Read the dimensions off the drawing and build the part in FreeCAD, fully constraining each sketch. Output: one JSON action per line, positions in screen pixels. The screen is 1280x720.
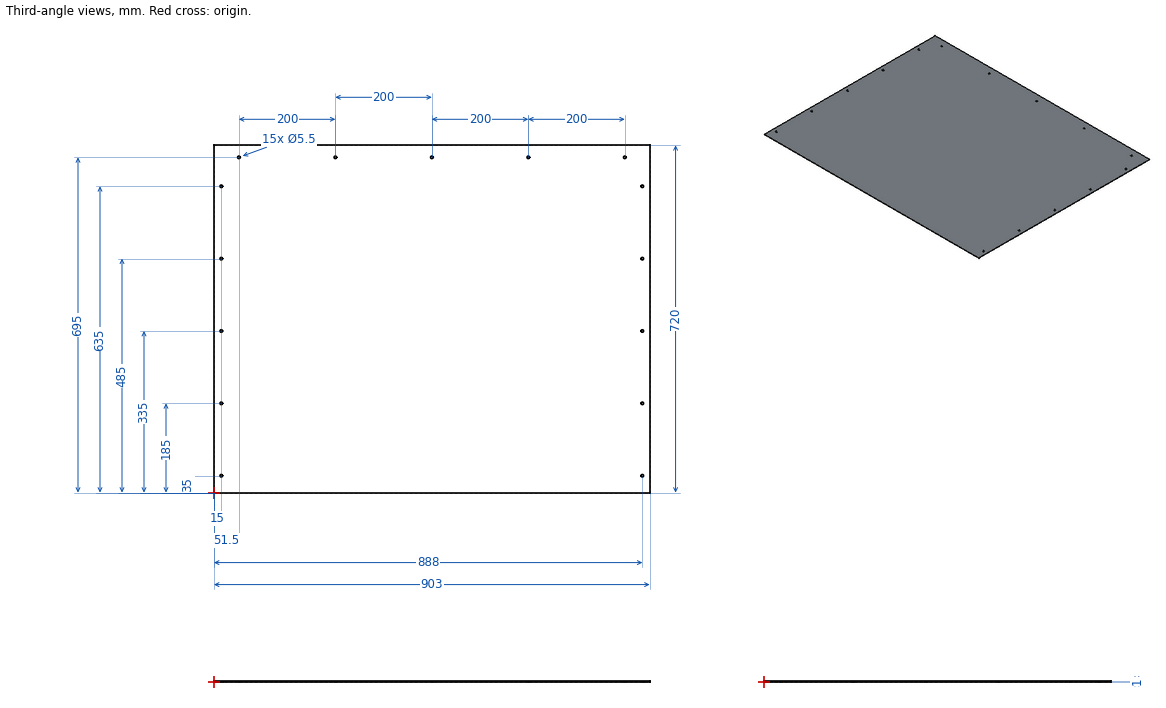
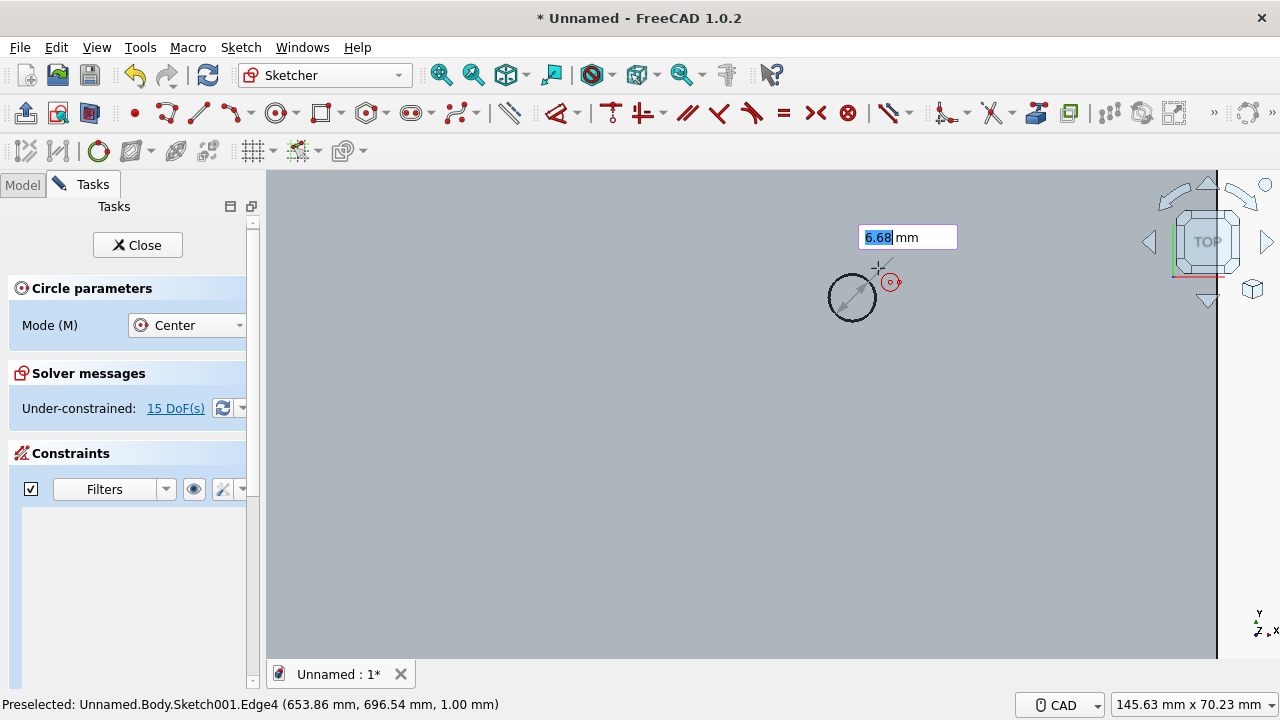
{"action": "left_click", "coordinate": [872, 260]}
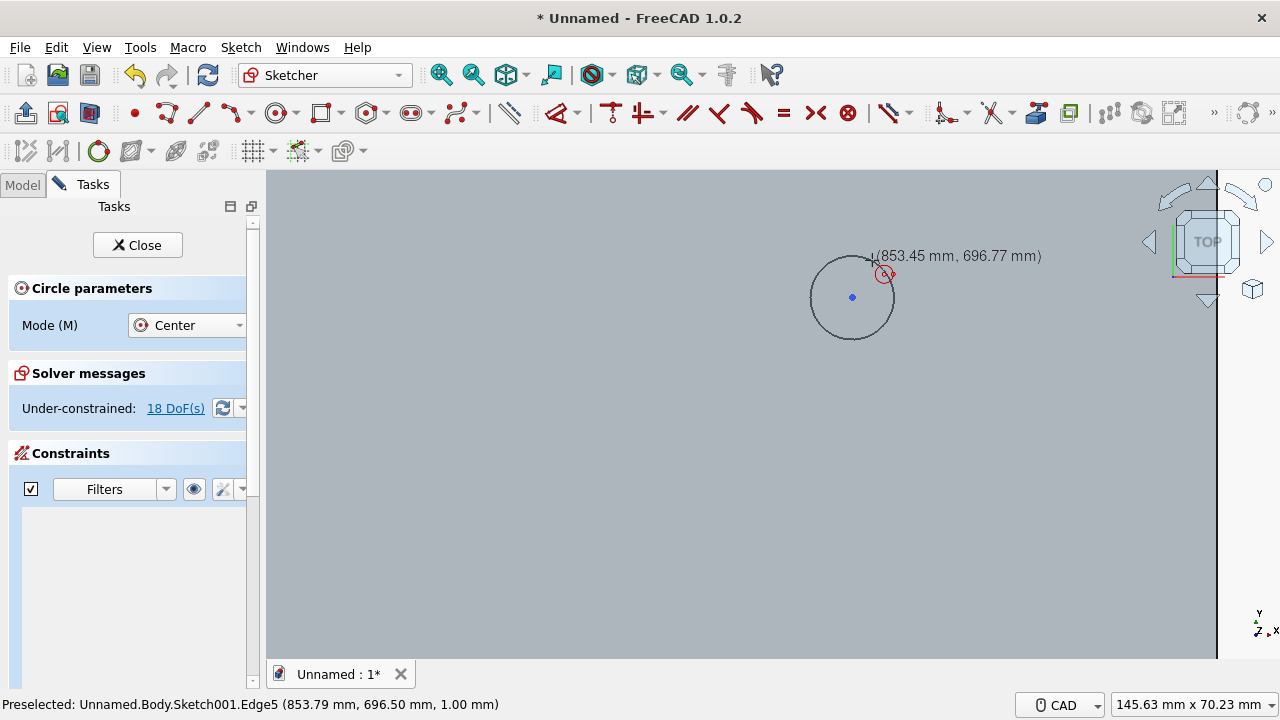
{"action": "scroll", "coordinate": [878, 268], "scroll_direction": "down", "scroll_amount": 14}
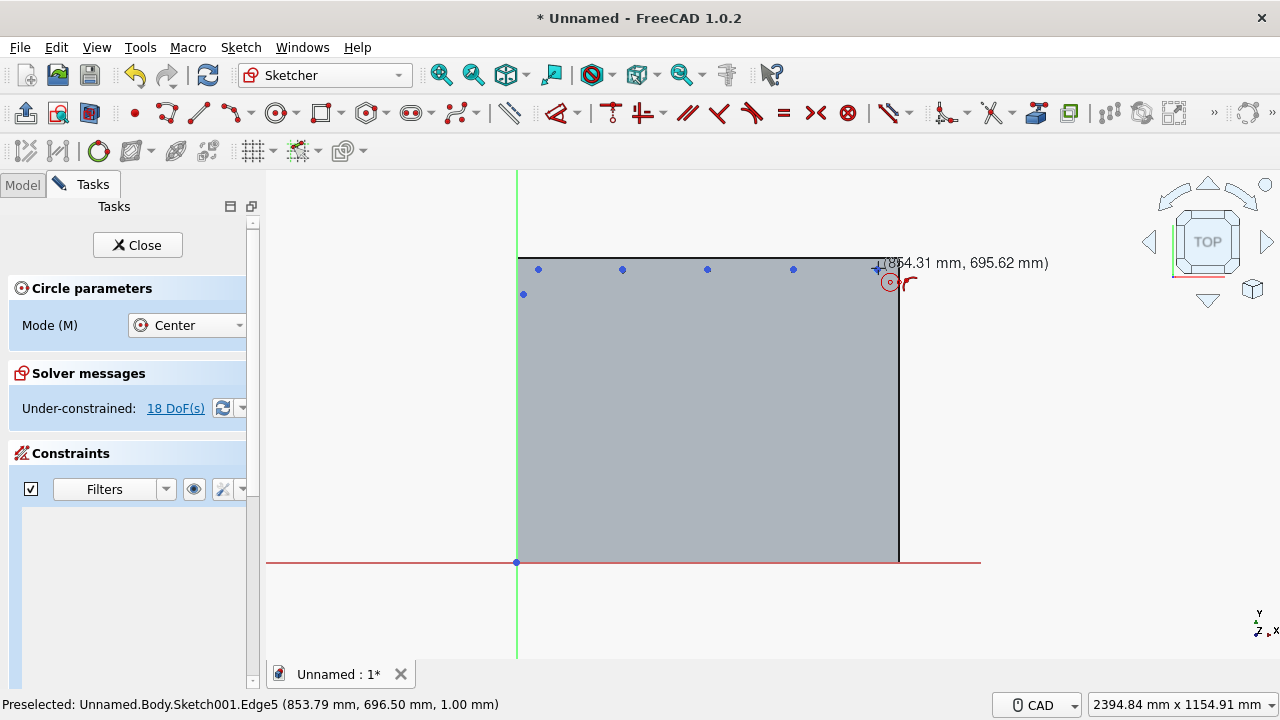
{"action": "scroll", "coordinate": [523, 357], "scroll_direction": "up", "scroll_amount": 15}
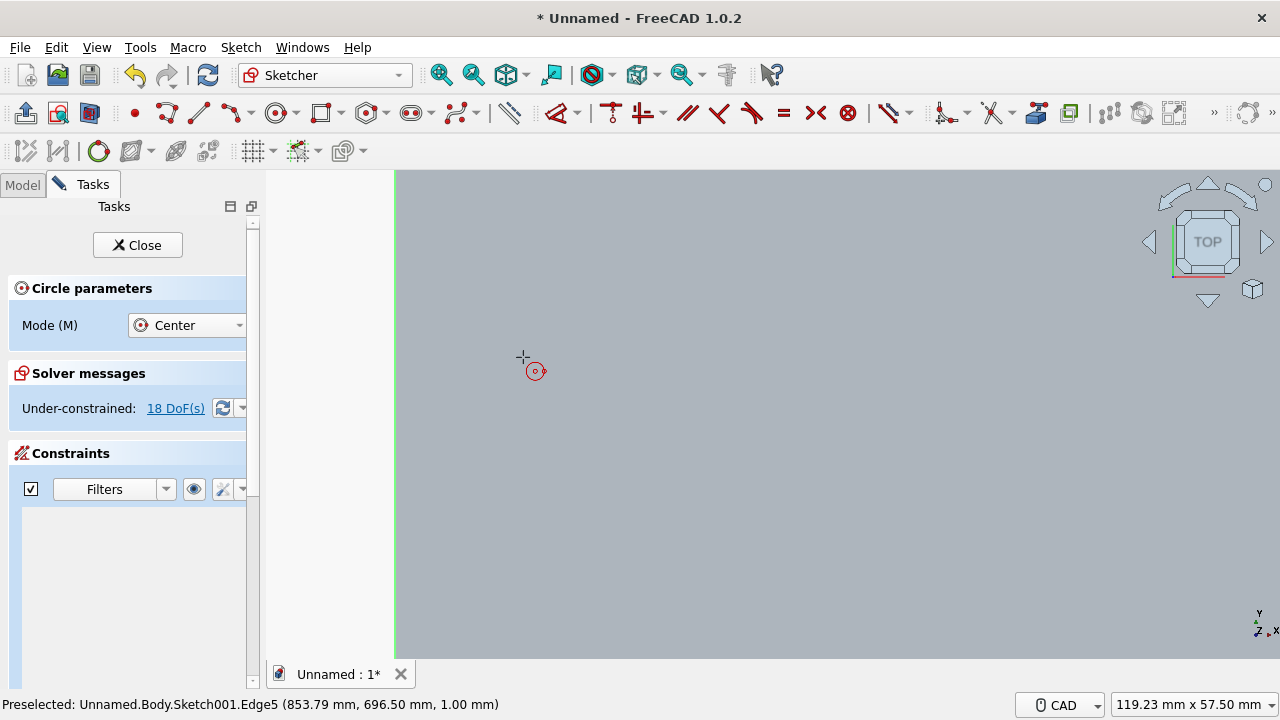
{"action": "scroll", "coordinate": [522, 357], "scroll_direction": "down", "scroll_amount": 15}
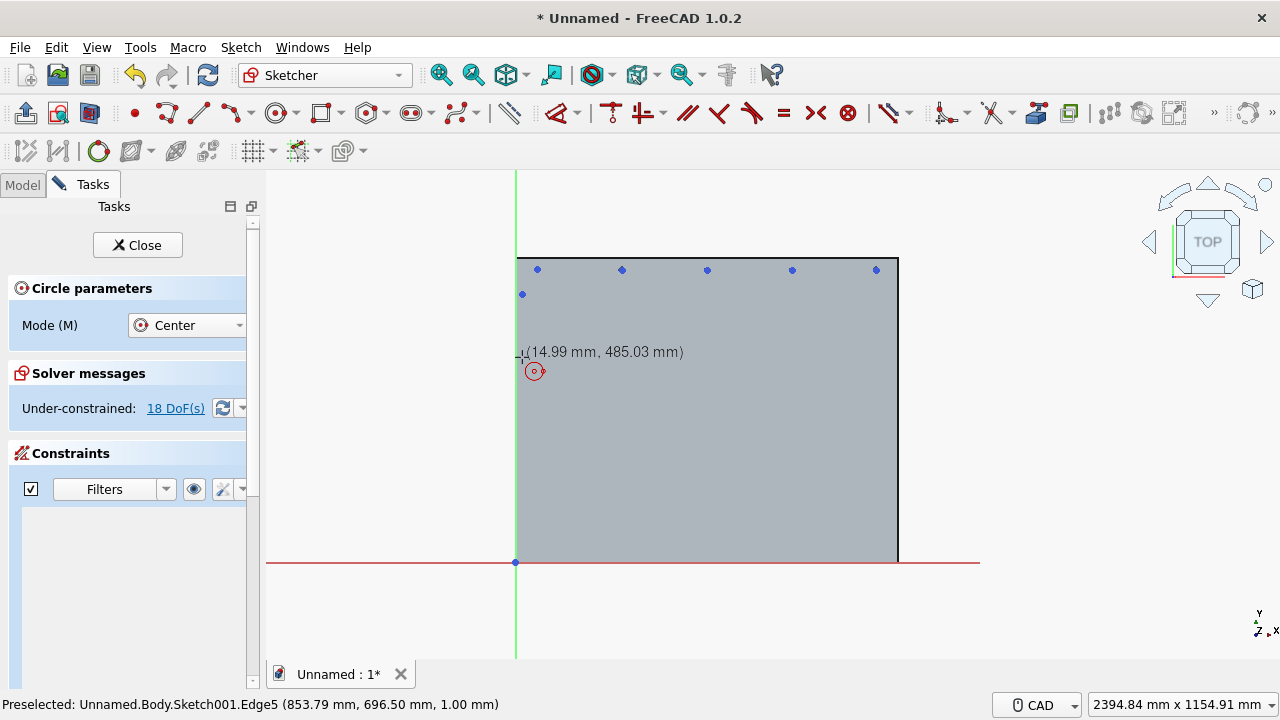
{"action": "scroll", "coordinate": [522, 357], "scroll_direction": "up", "scroll_amount": 5}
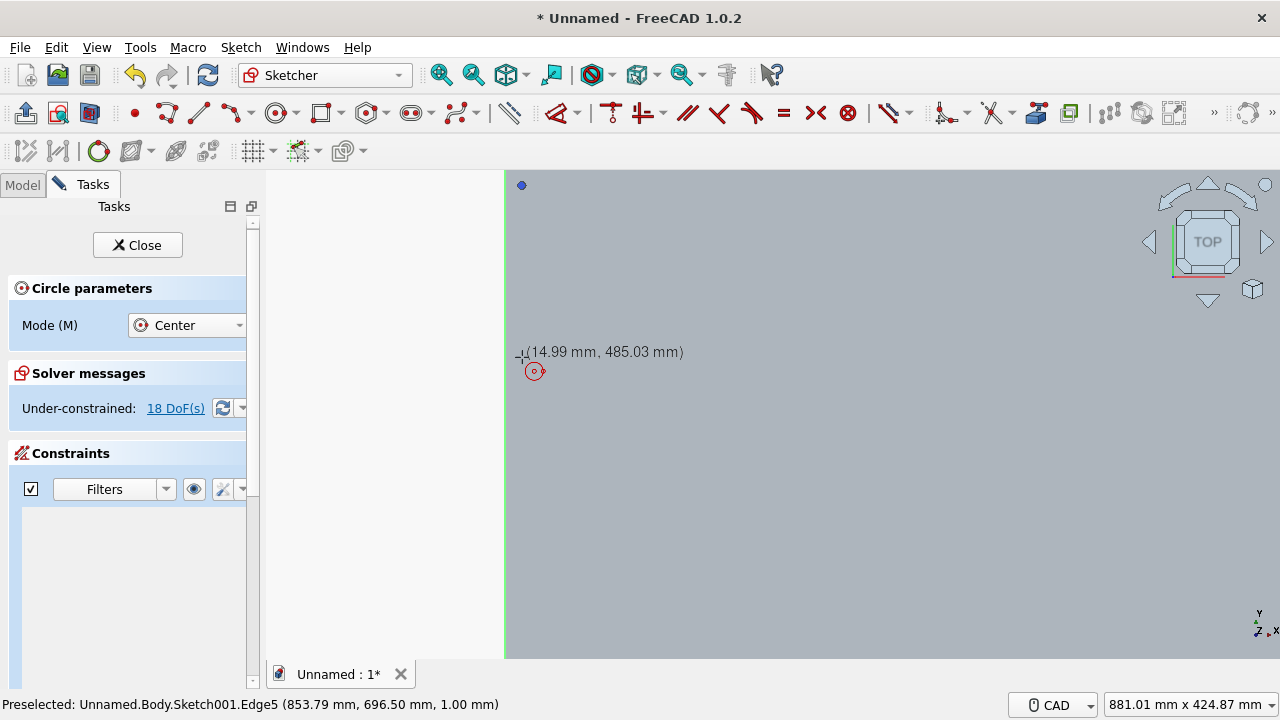
{"action": "left_click", "coordinate": [522, 358]}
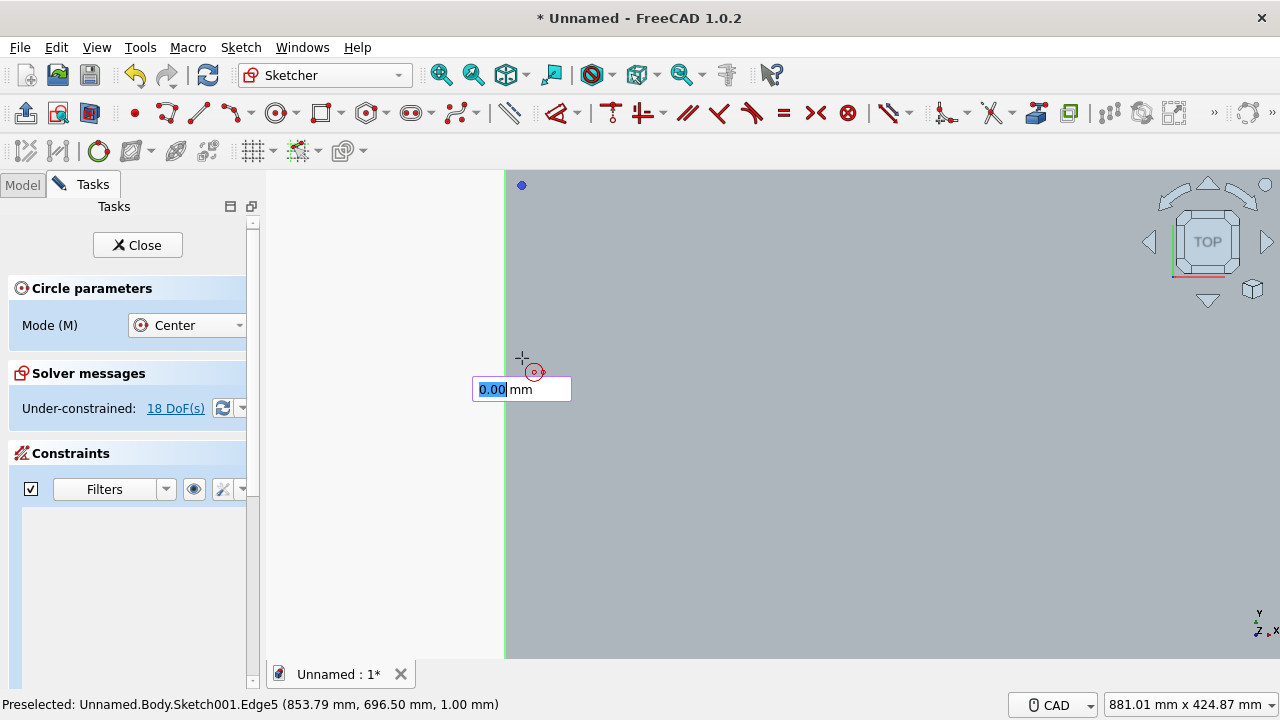
{"action": "scroll", "coordinate": [524, 355], "scroll_direction": "up", "scroll_amount": 9}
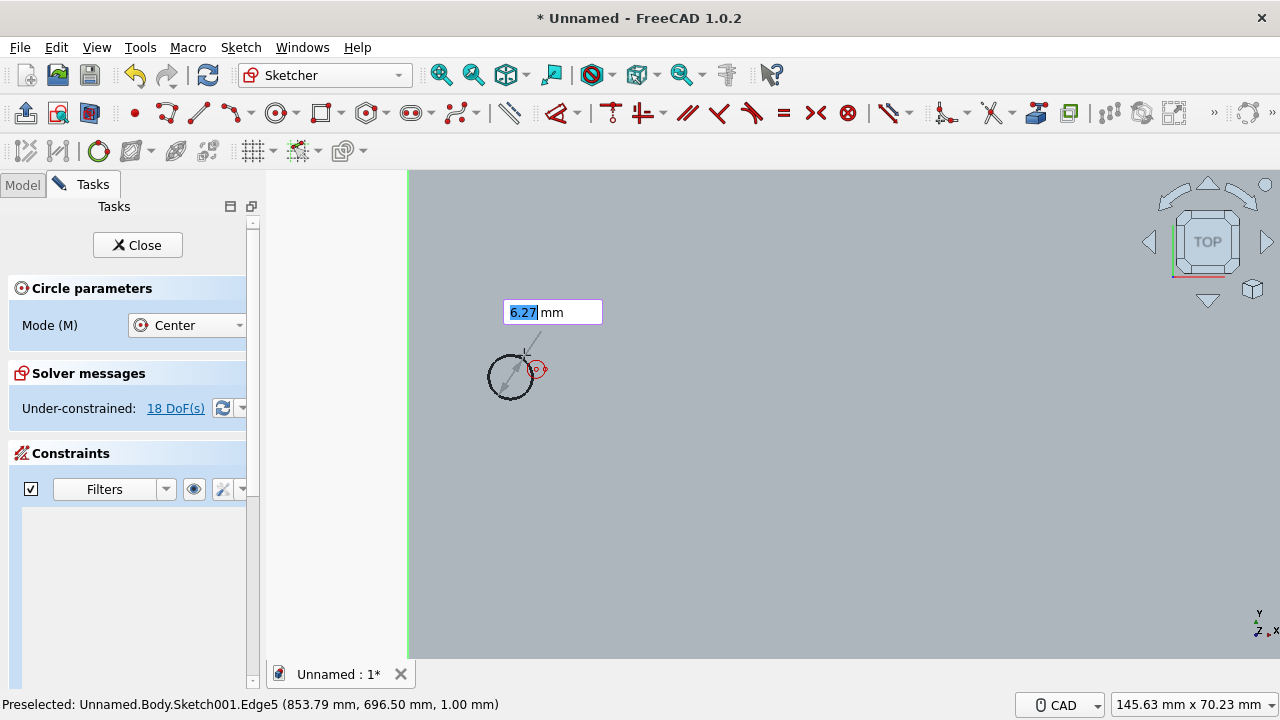
{"action": "left_click", "coordinate": [526, 355]}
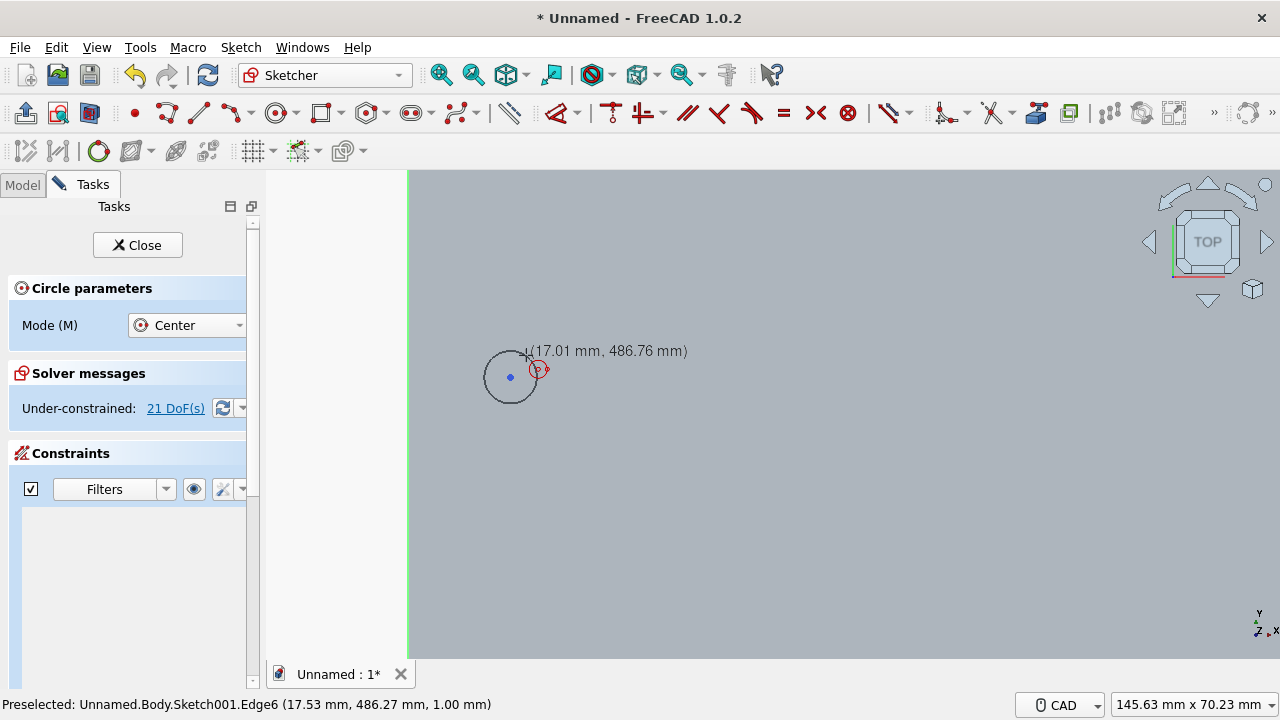
{"action": "scroll", "coordinate": [523, 356], "scroll_direction": "down", "scroll_amount": 14}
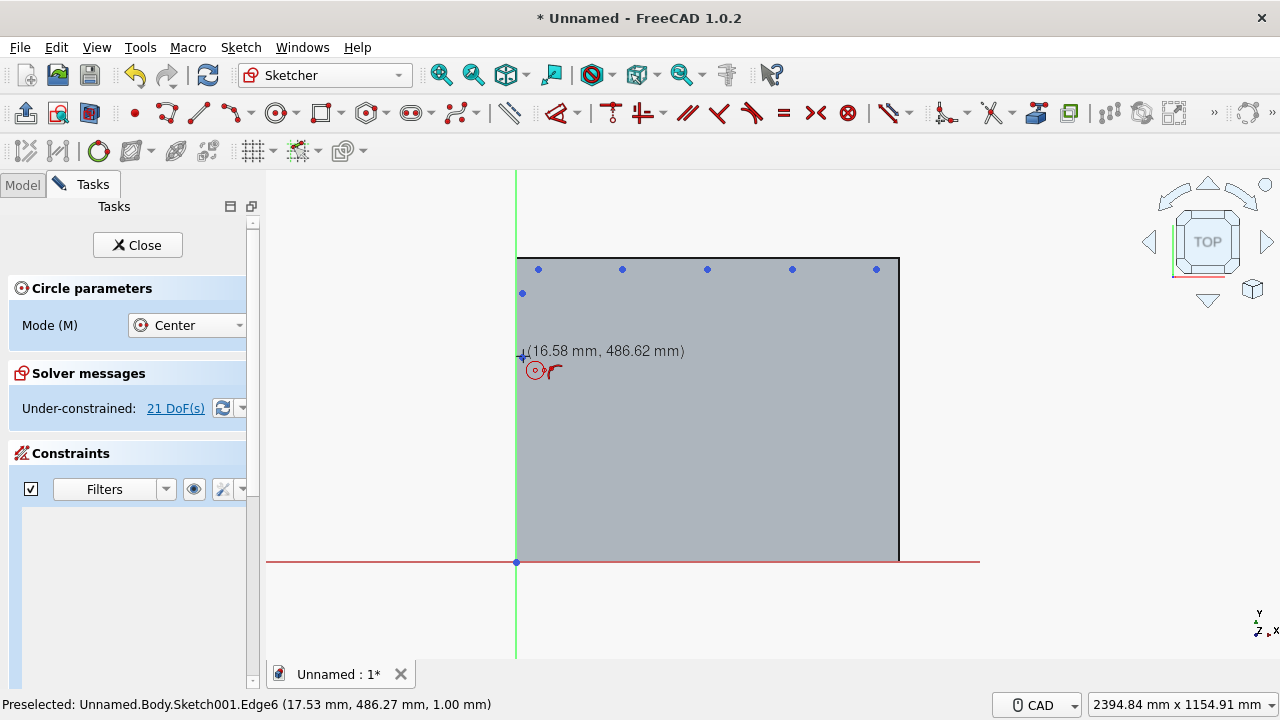
{"action": "scroll", "coordinate": [523, 421], "scroll_direction": "up", "scroll_amount": 15}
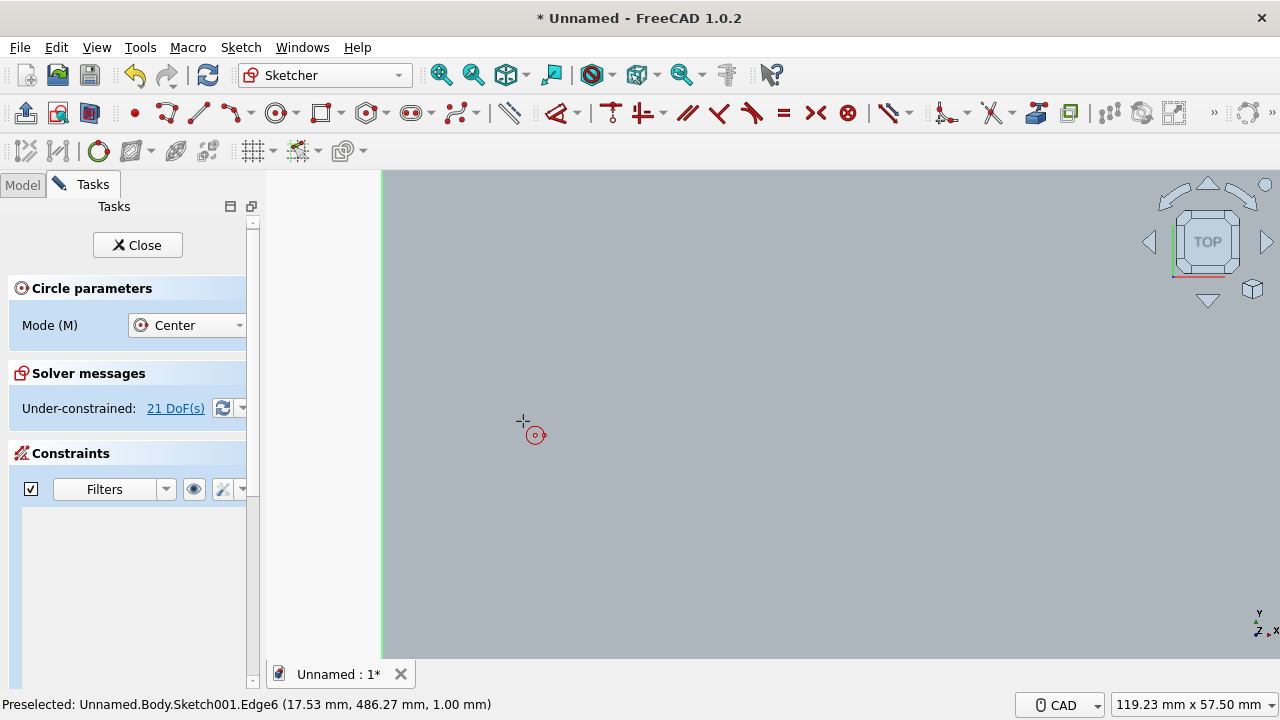
{"action": "scroll", "coordinate": [523, 421], "scroll_direction": "down", "scroll_amount": 15}